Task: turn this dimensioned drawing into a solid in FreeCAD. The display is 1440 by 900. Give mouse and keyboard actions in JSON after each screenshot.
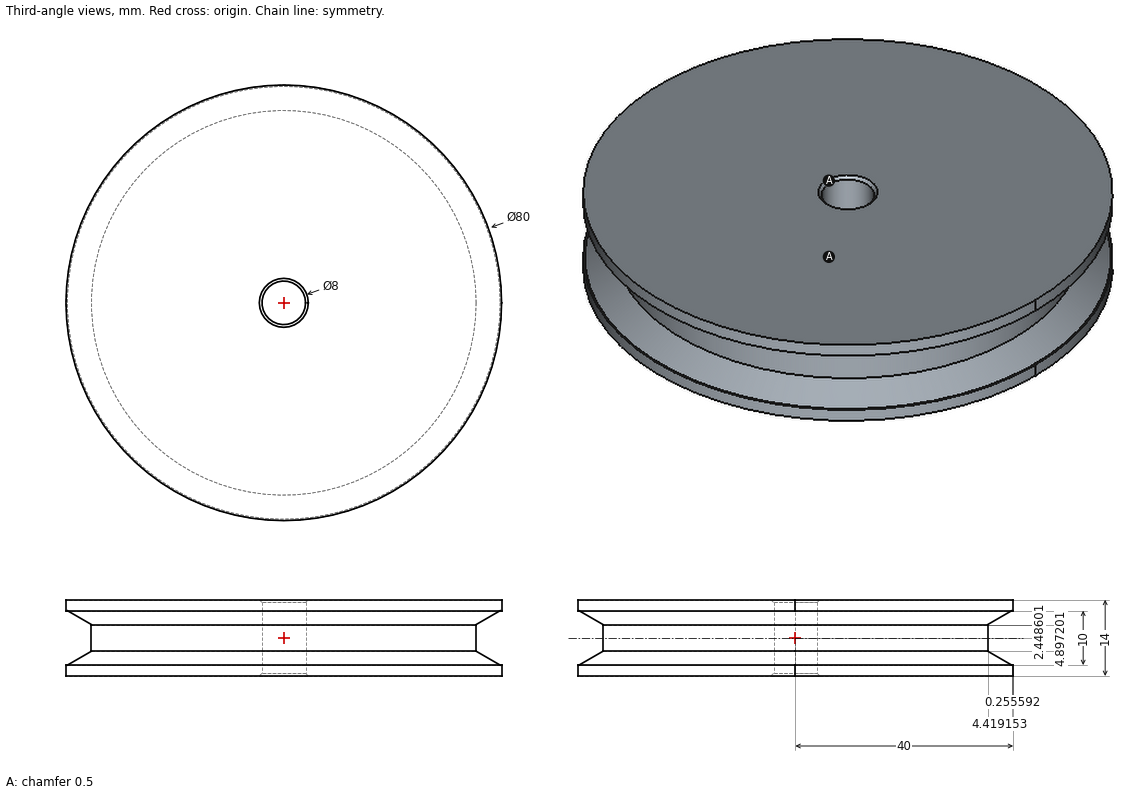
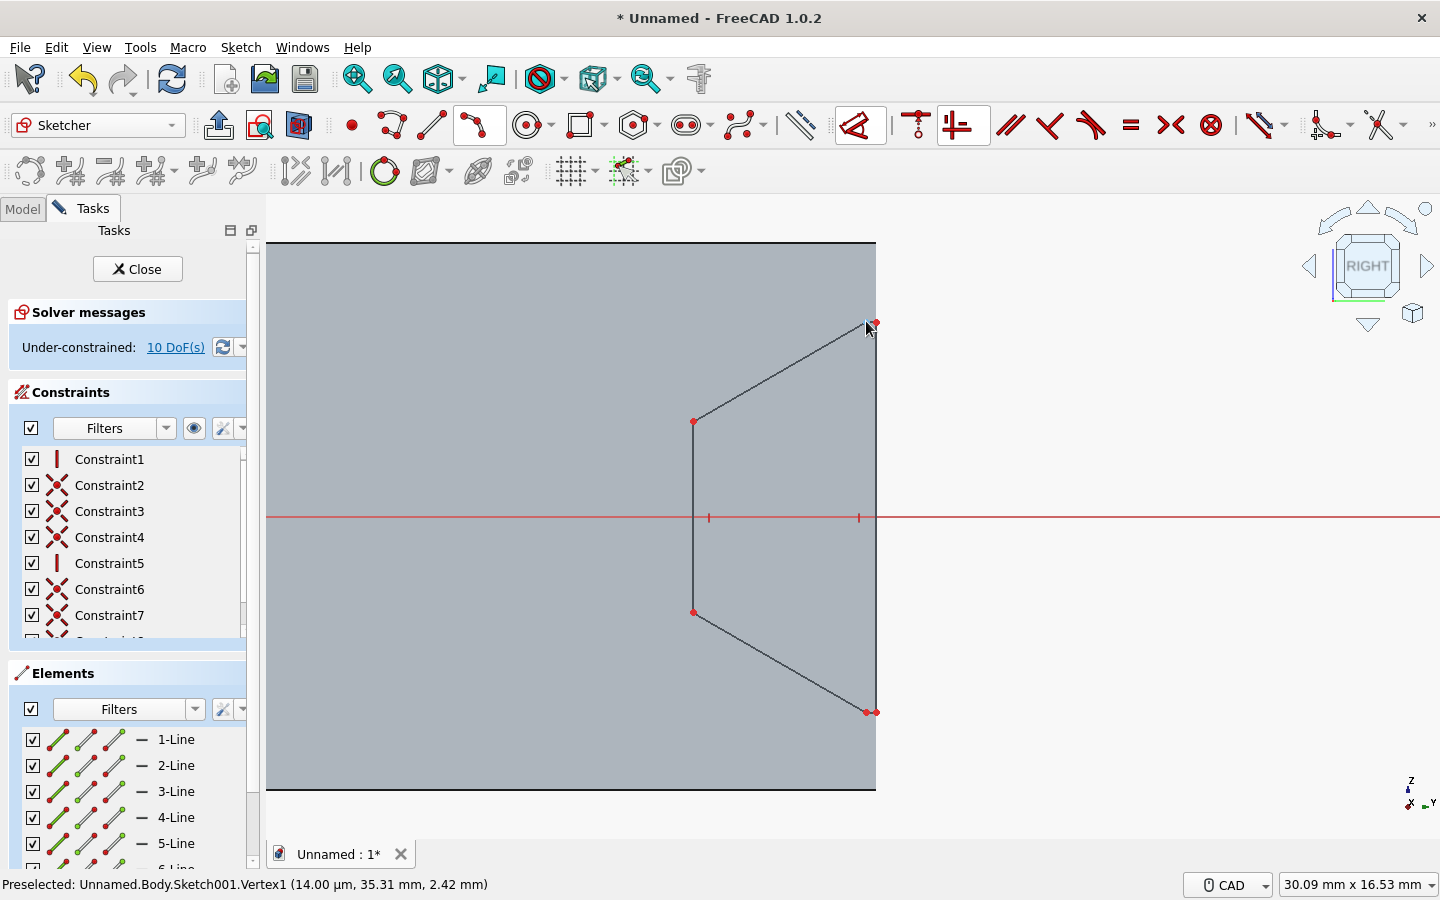
{"action": "scroll", "coordinate": [871, 713], "scroll_direction": "up", "scroll_amount": 6}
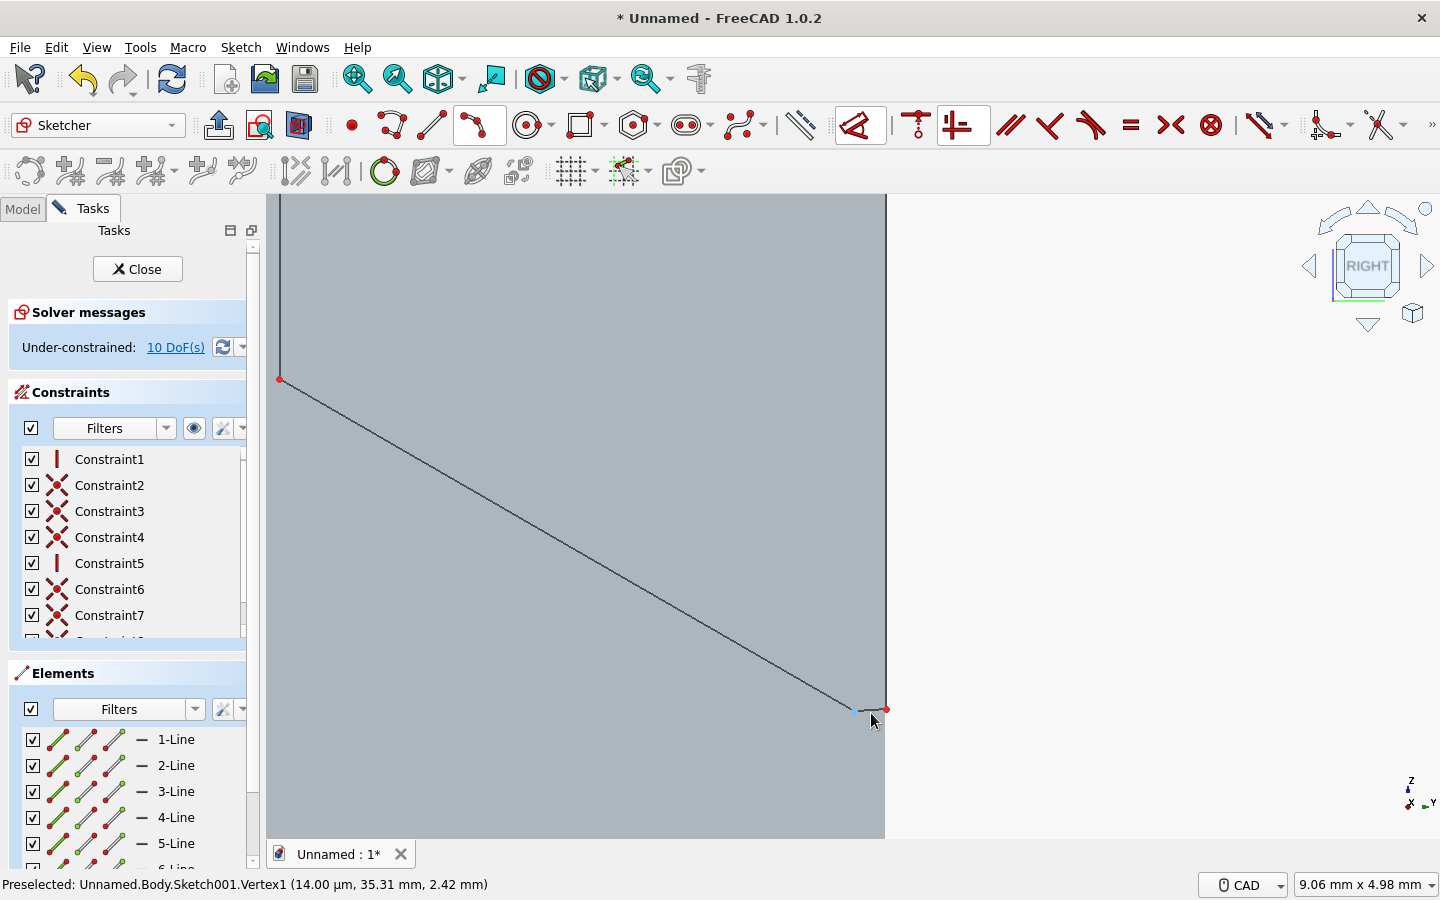
{"action": "left_click", "coordinate": [870, 710]}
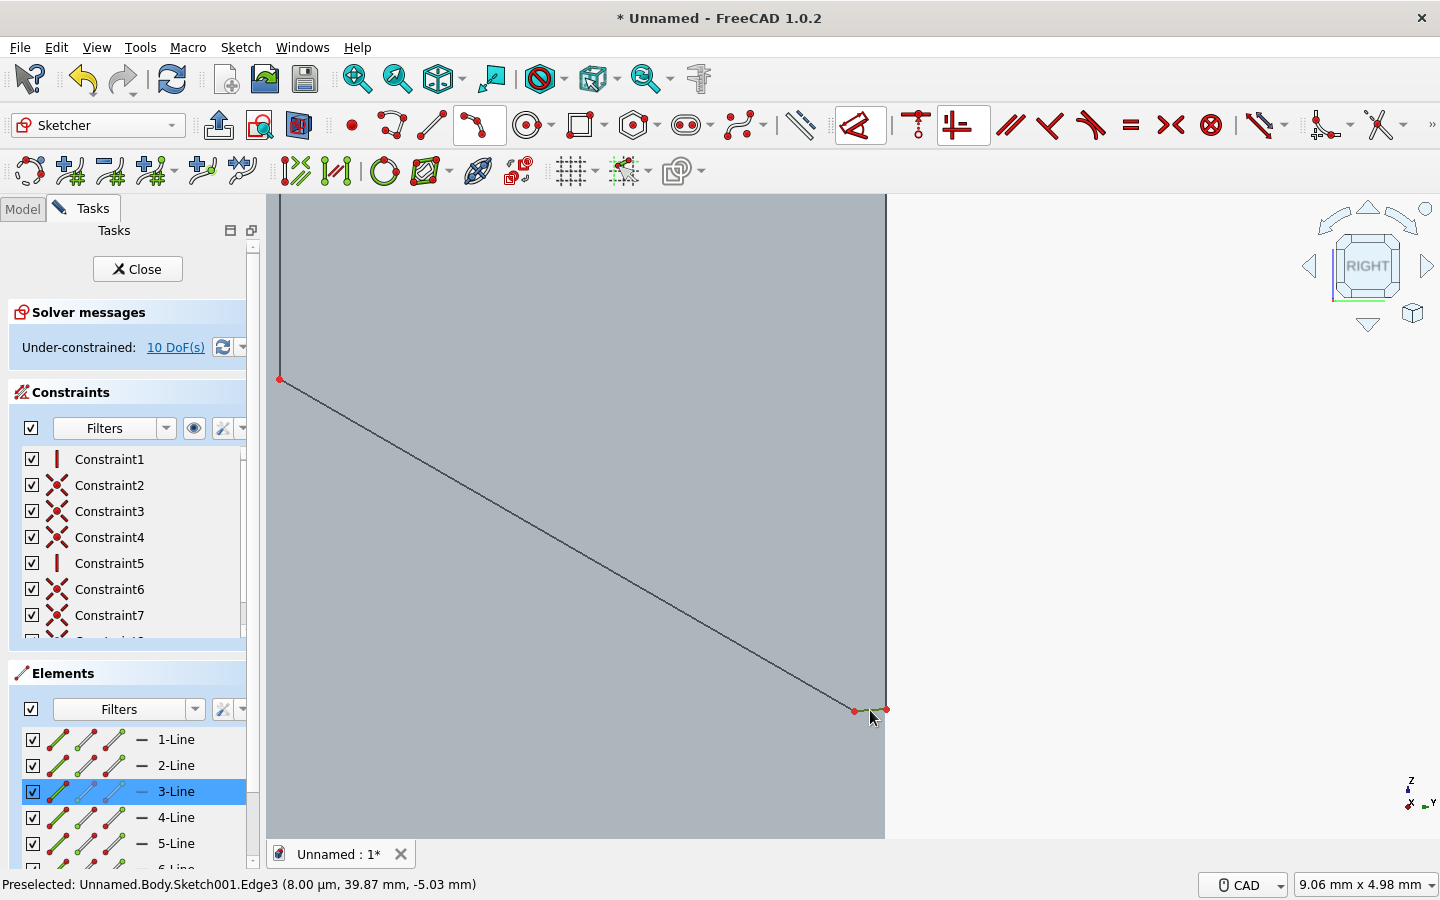
{"action": "left_click", "coordinate": [984, 126]}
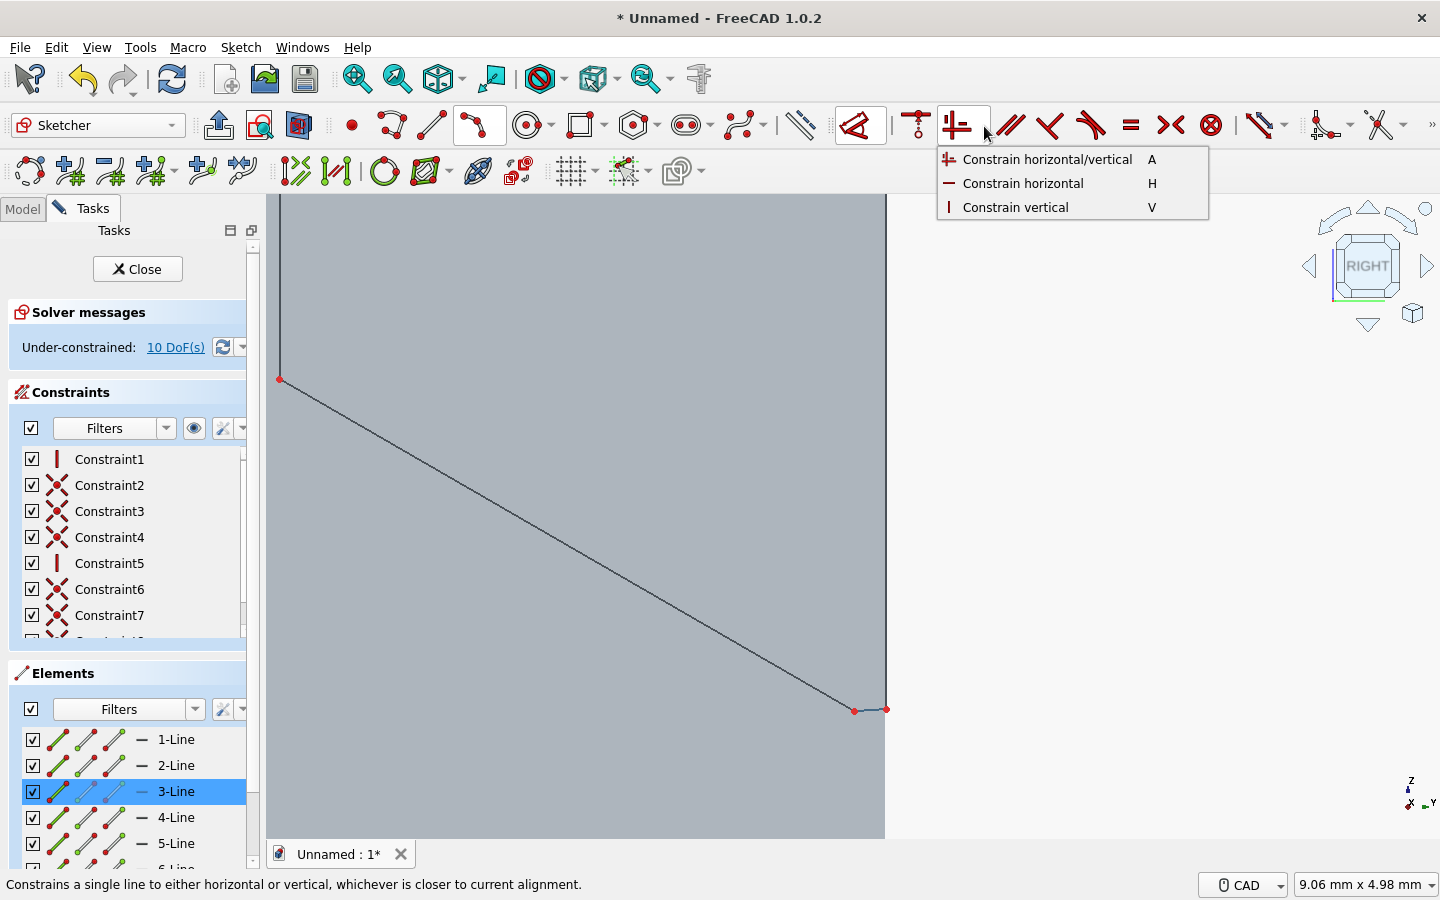
{"action": "left_click", "coordinate": [1073, 183]}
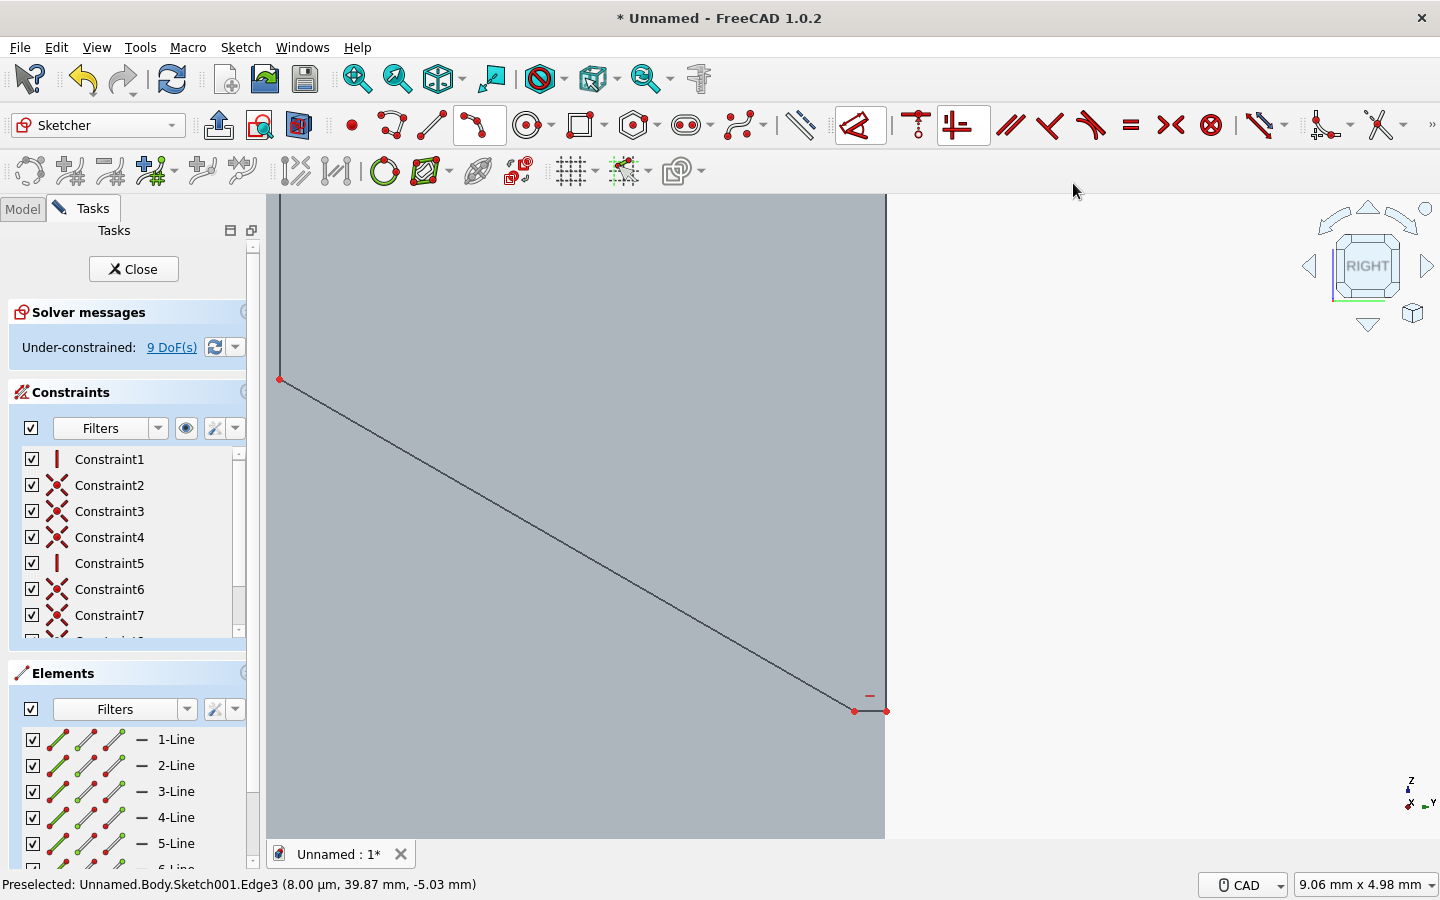
{"action": "scroll", "coordinate": [871, 714], "scroll_direction": "down", "scroll_amount": 6}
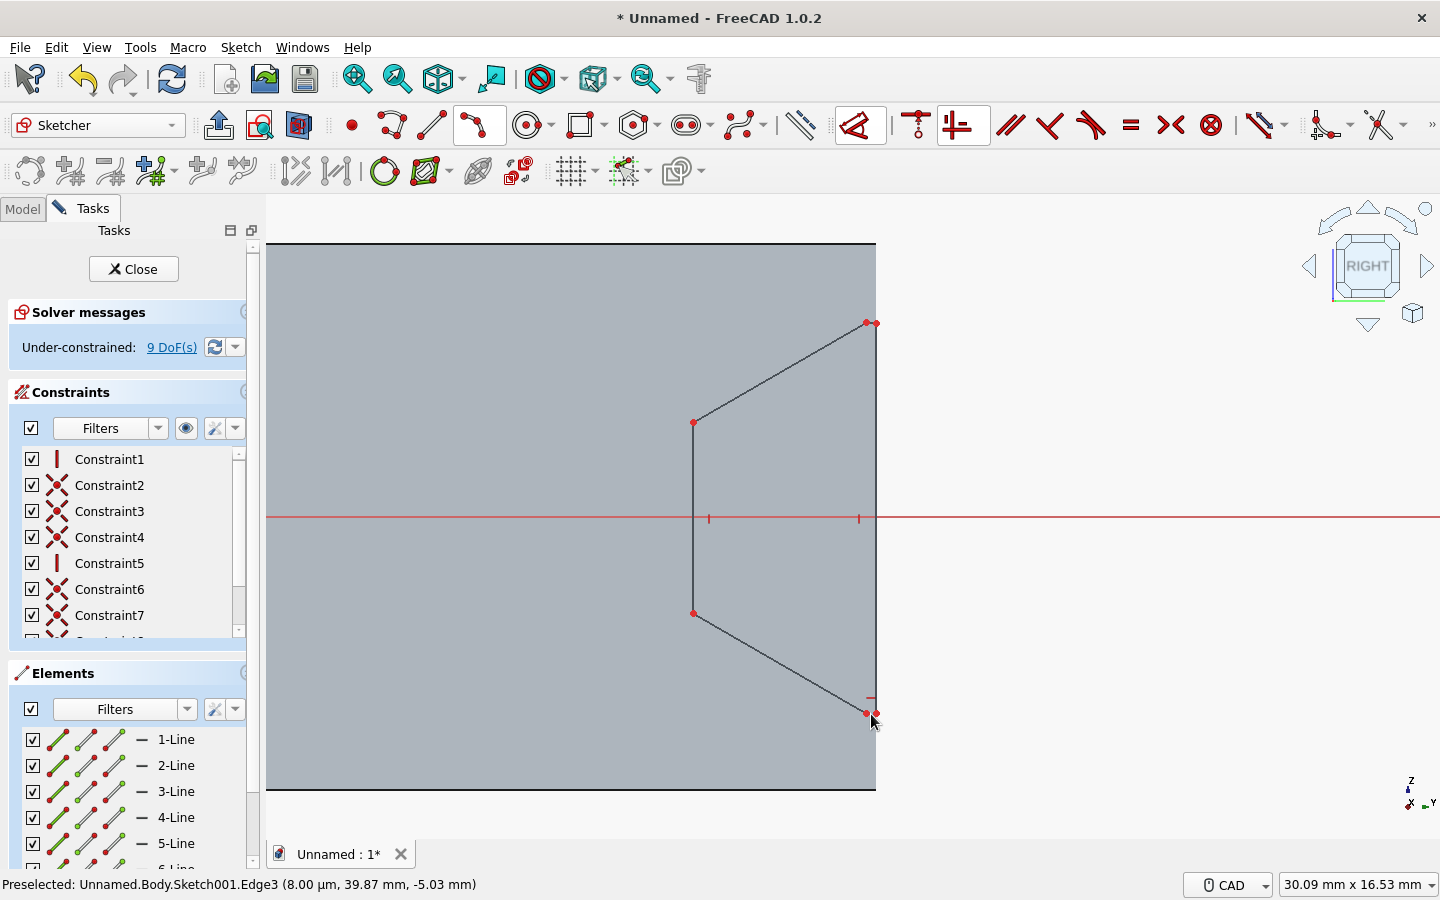
{"action": "scroll", "coordinate": [873, 323], "scroll_direction": "up", "scroll_amount": 8}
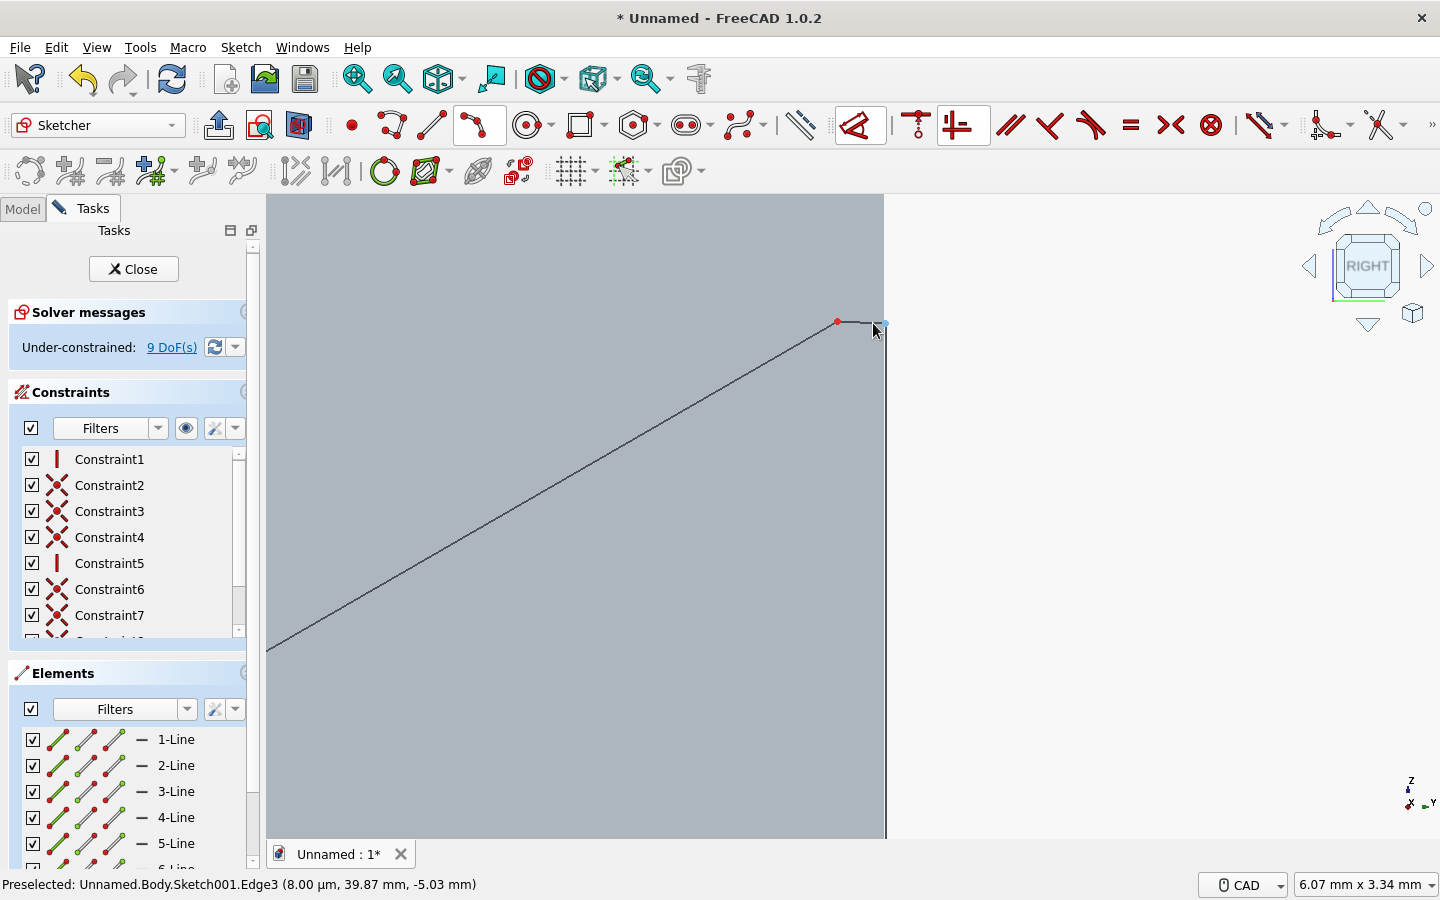
{"action": "left_click", "coordinate": [871, 323]}